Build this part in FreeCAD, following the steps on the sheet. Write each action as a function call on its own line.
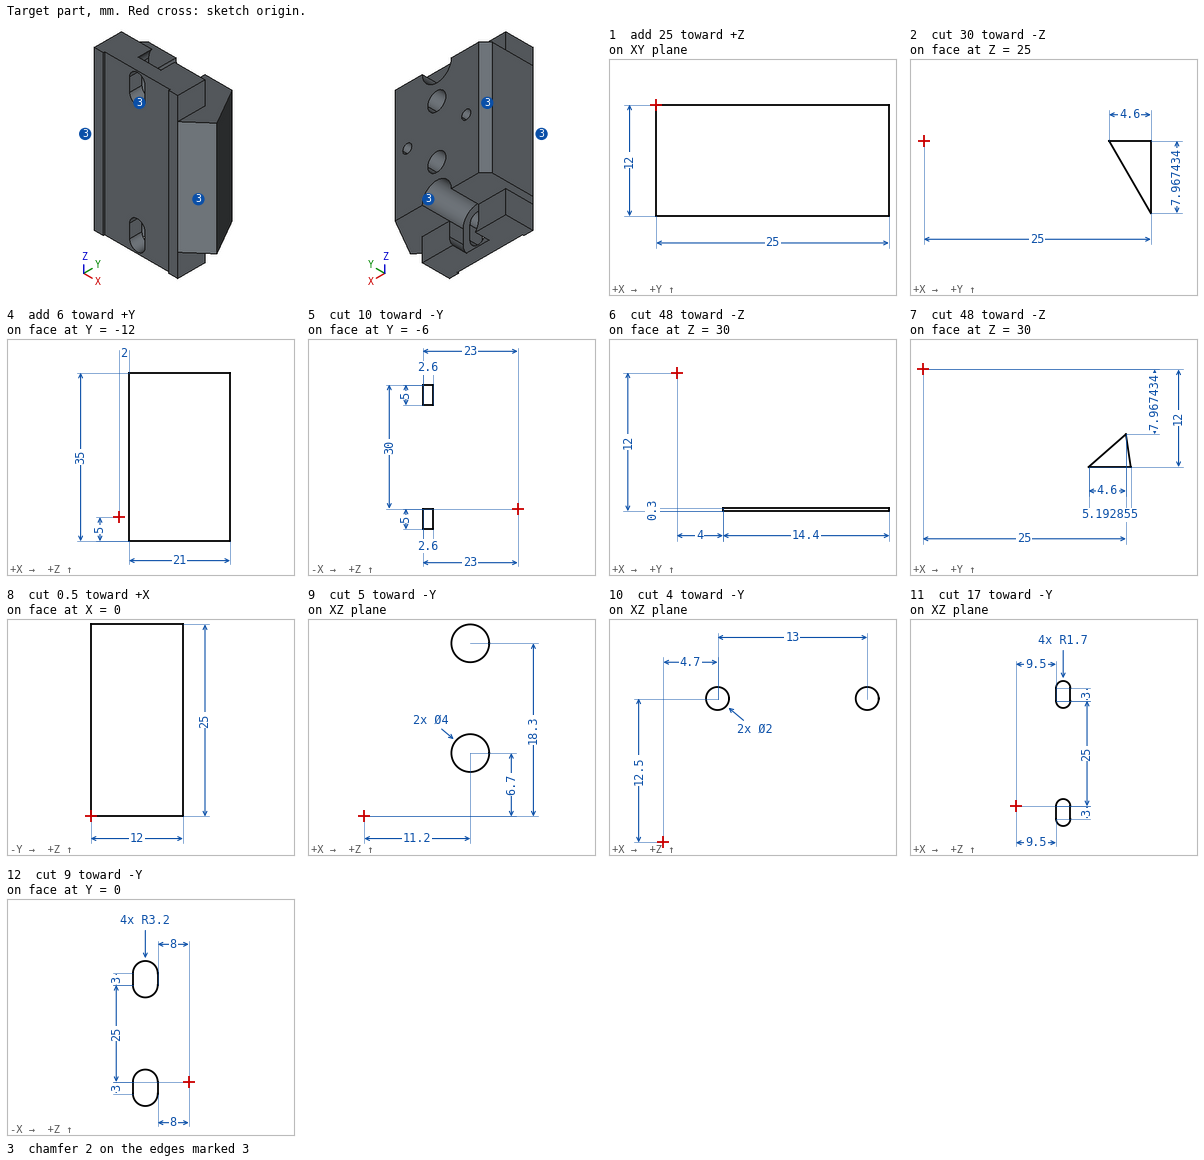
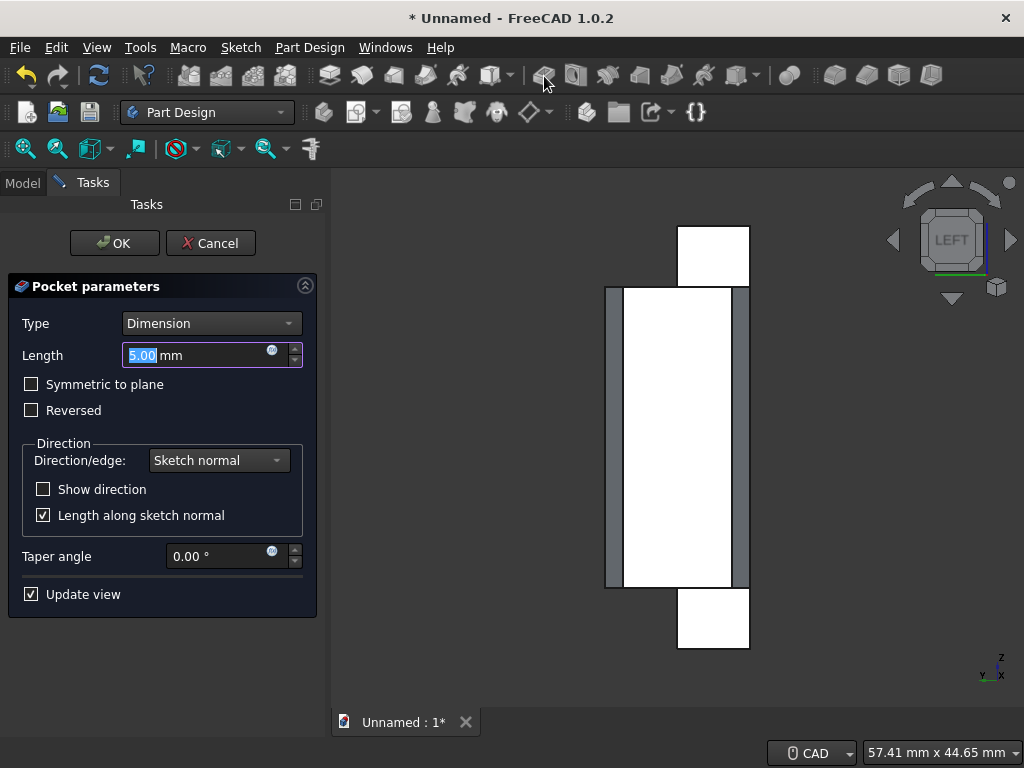
text(17)
key(Tab)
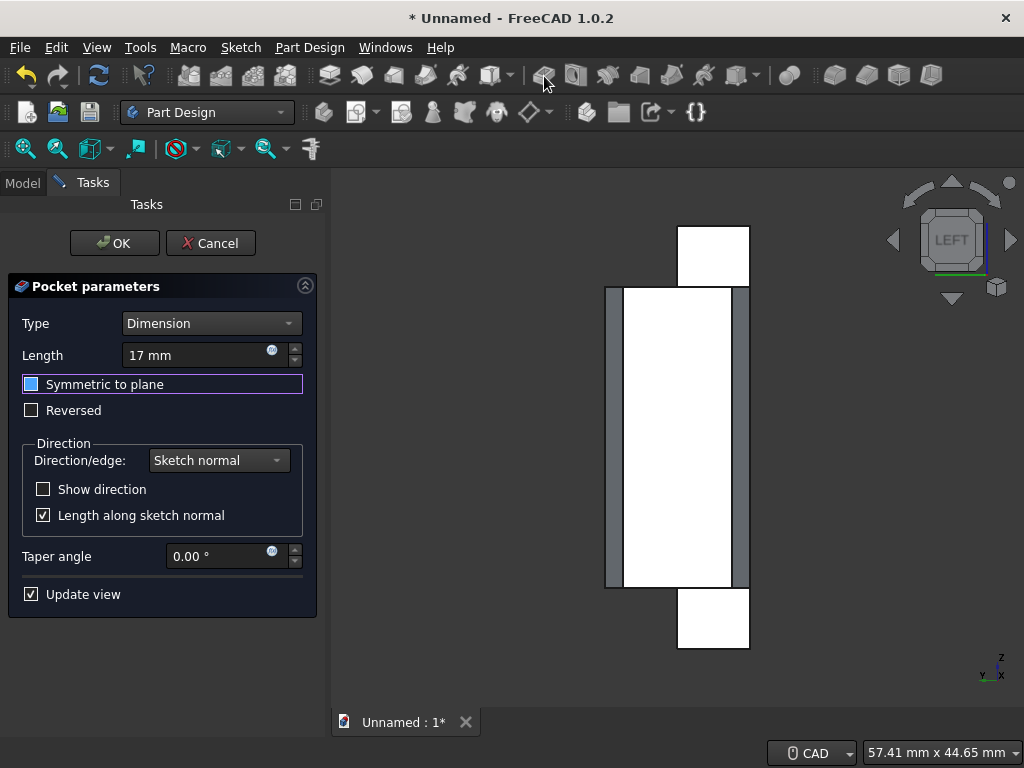
click(30, 410)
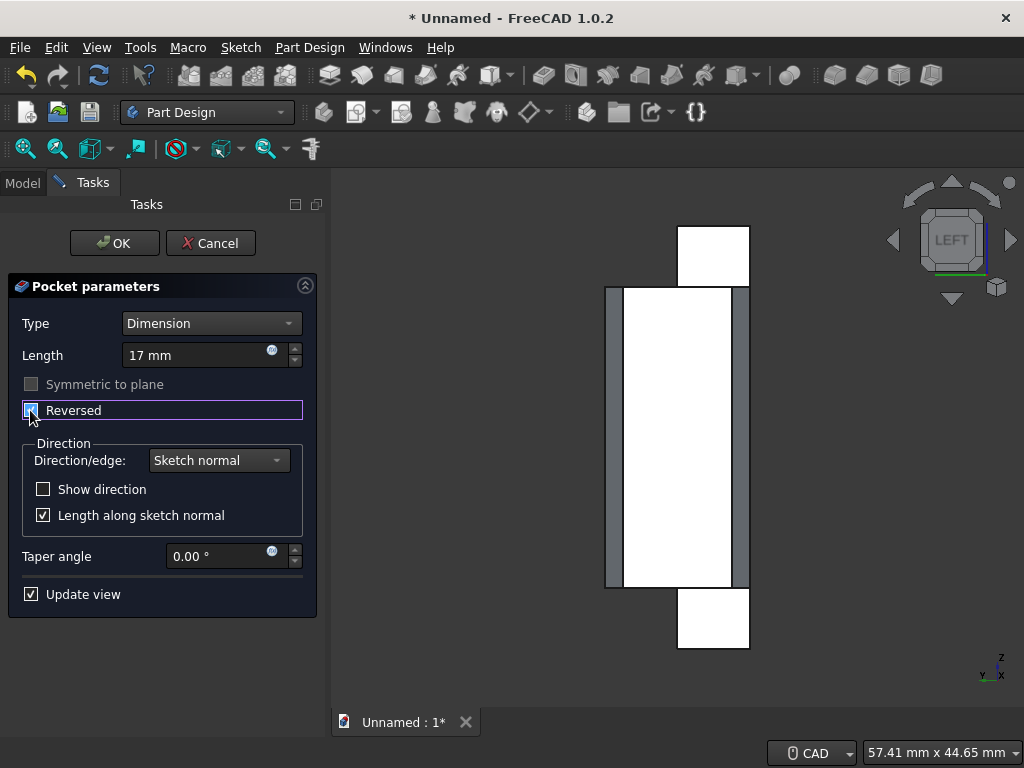
click(115, 243)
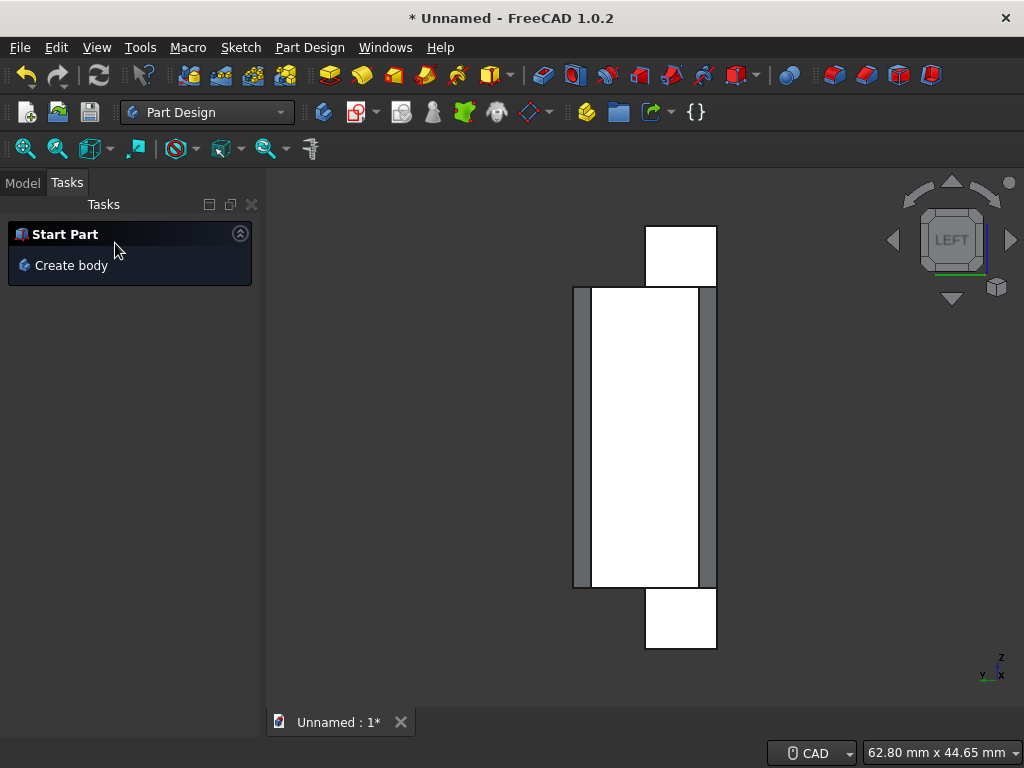
key(4)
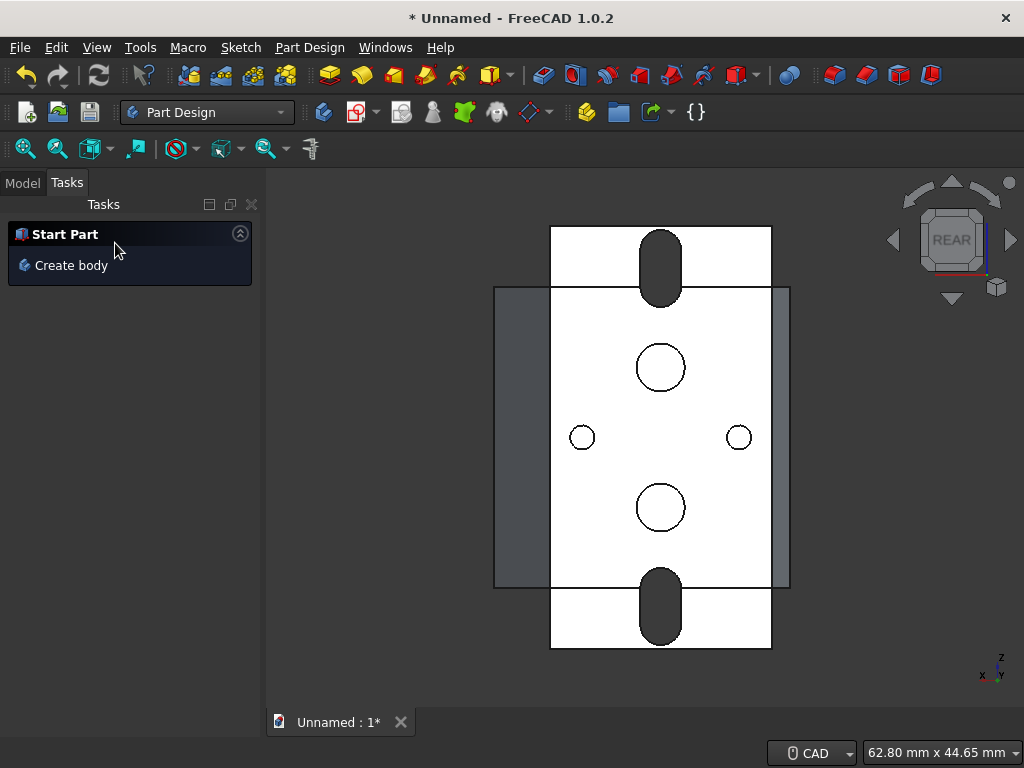
click(661, 437)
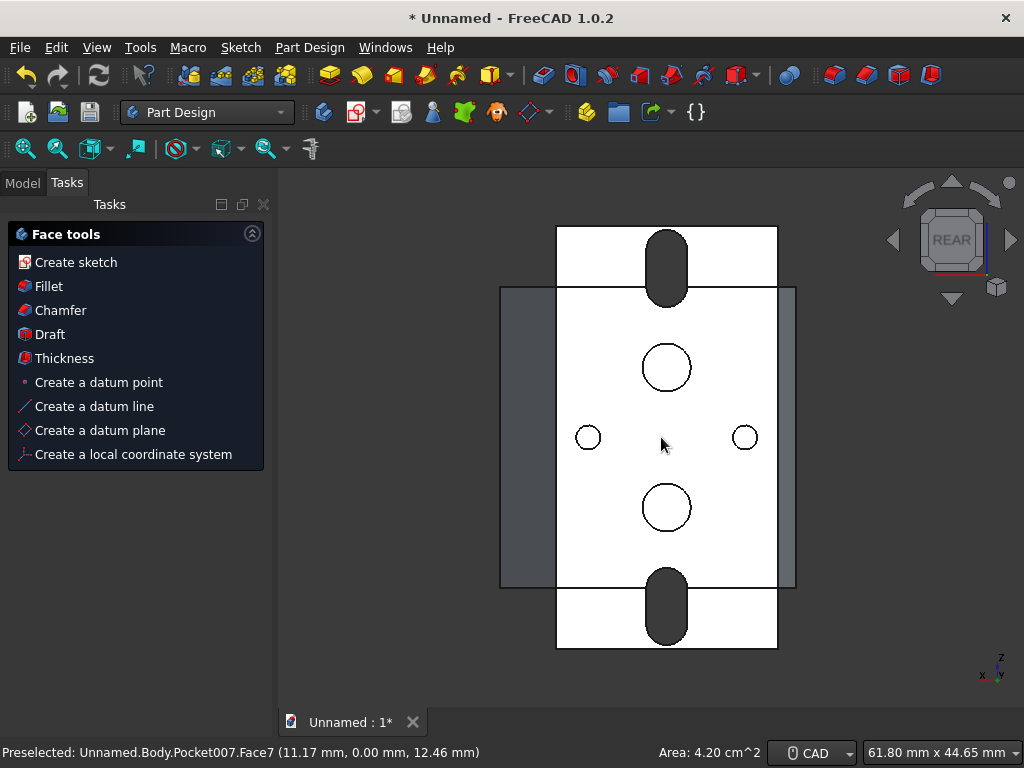
click(356, 112)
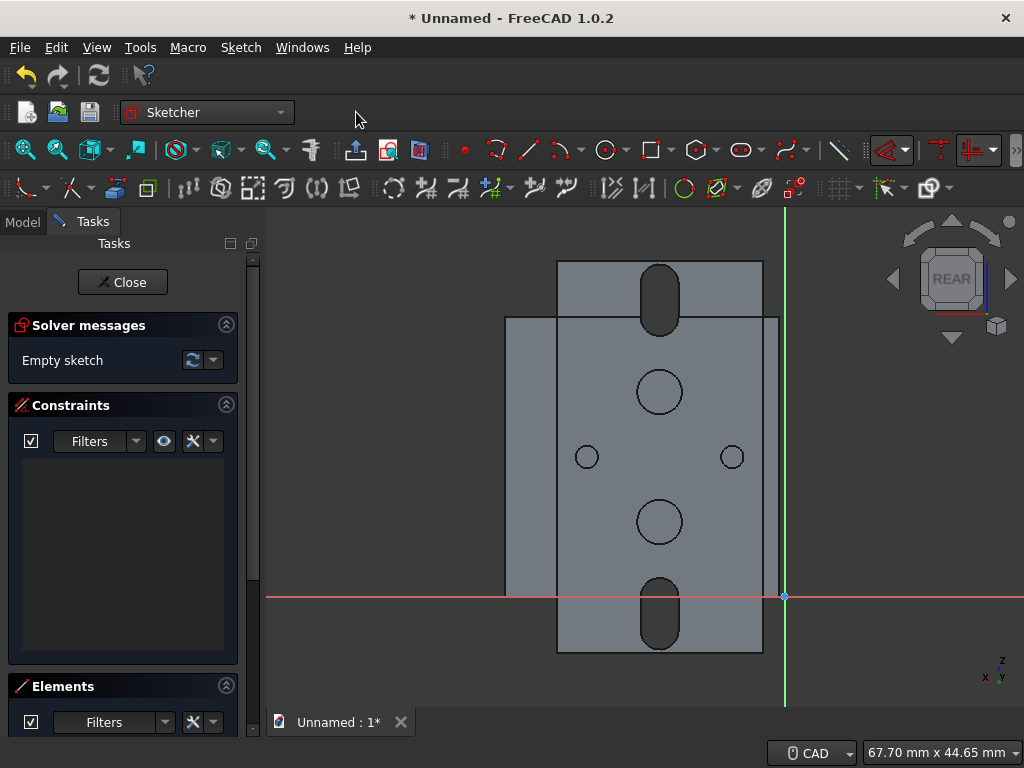
scroll(294, 457, down, 1)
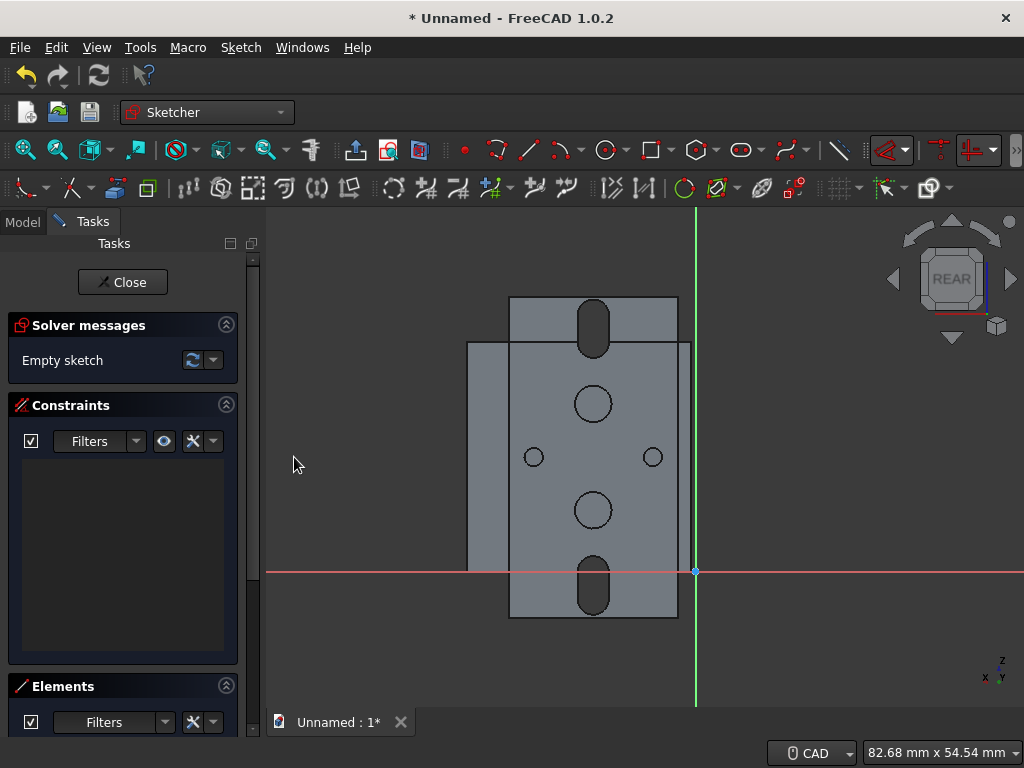
click(742, 150)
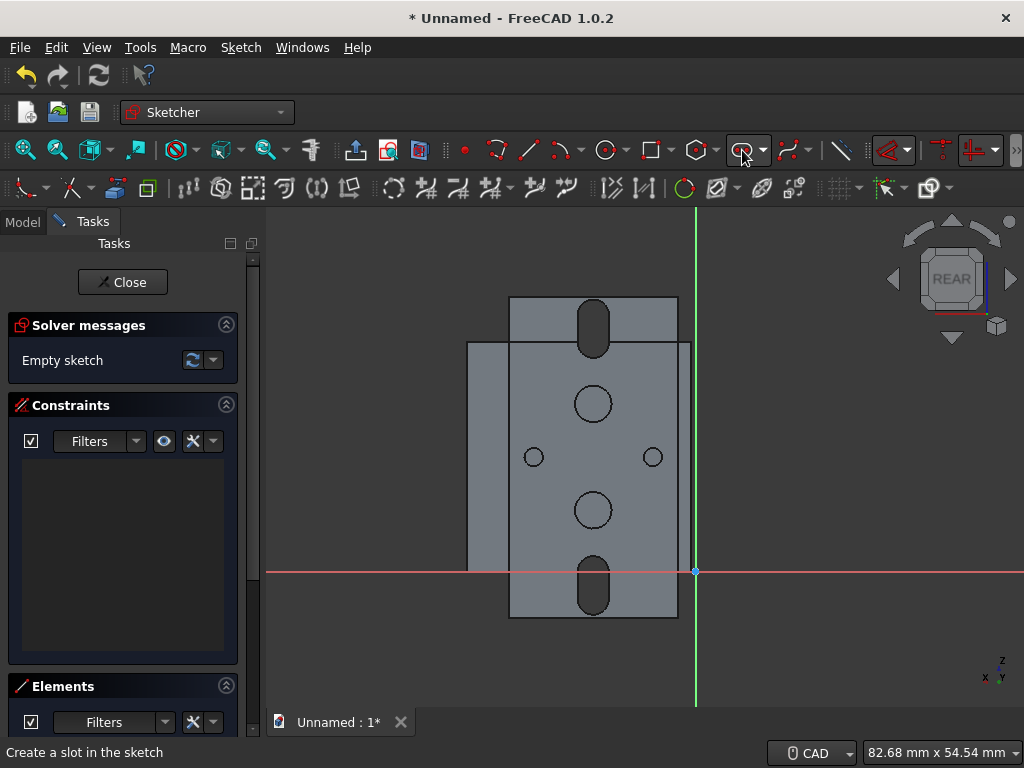
click(593, 342)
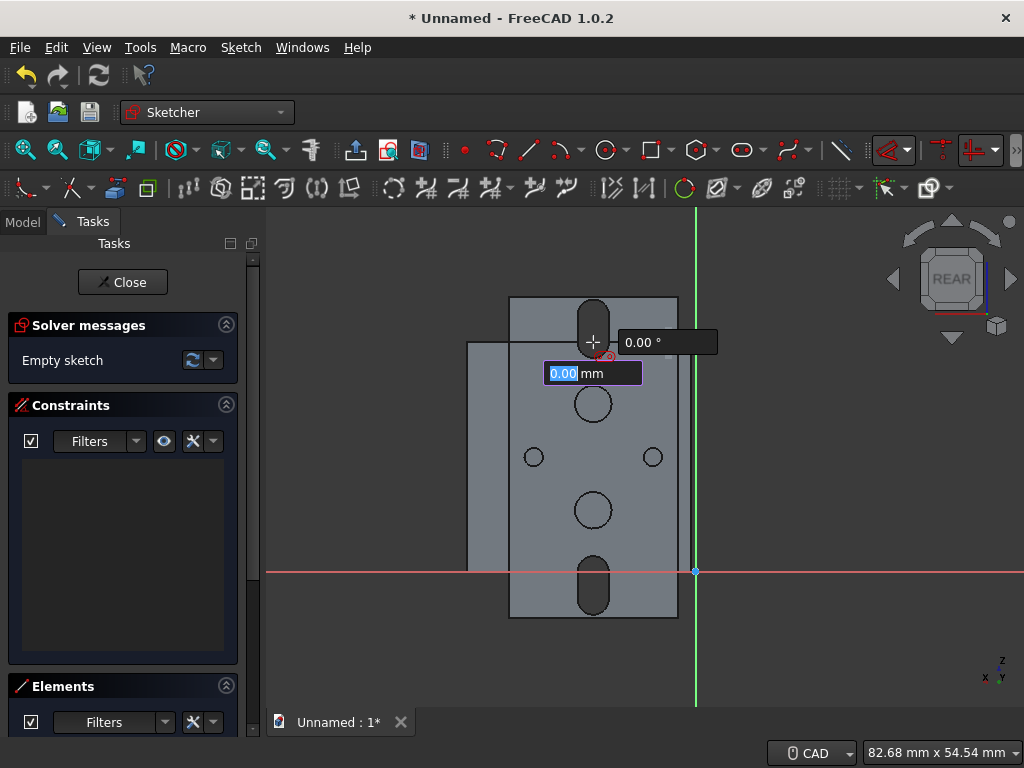
click(593, 315)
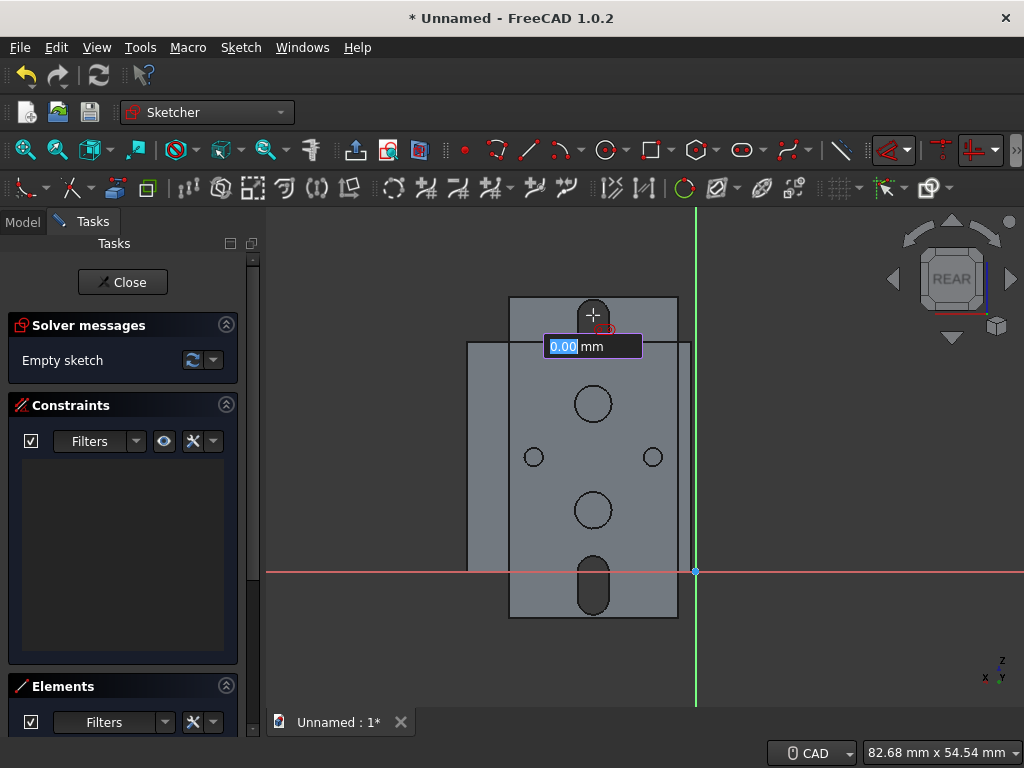
click(564, 329)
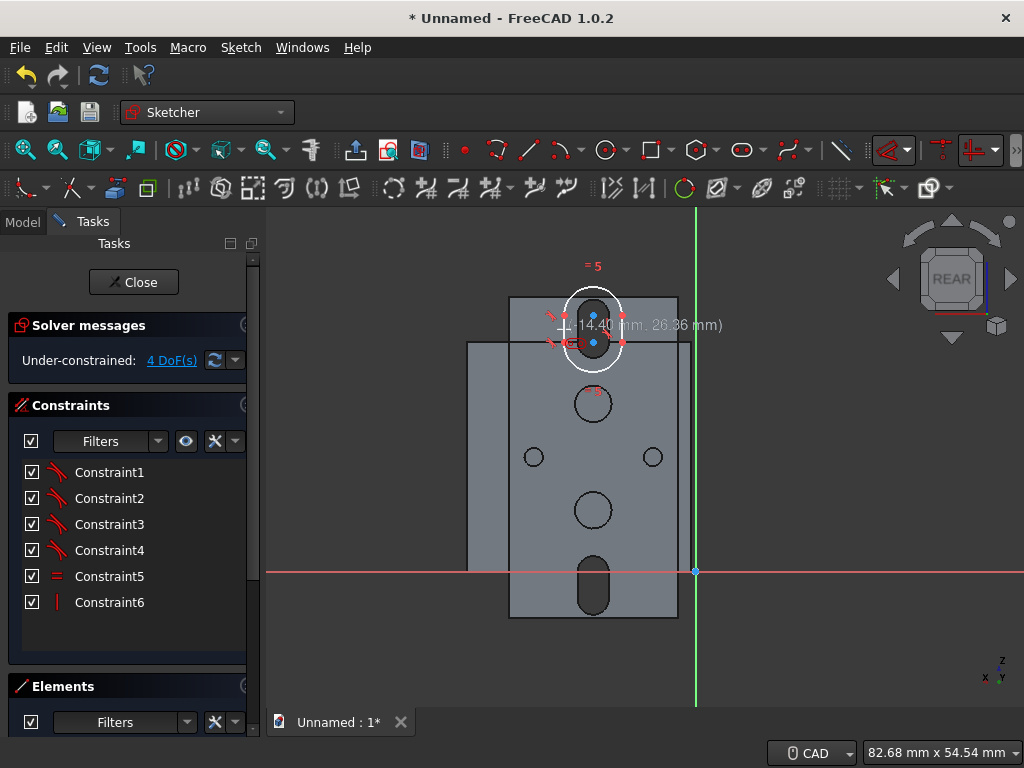
click(593, 599)